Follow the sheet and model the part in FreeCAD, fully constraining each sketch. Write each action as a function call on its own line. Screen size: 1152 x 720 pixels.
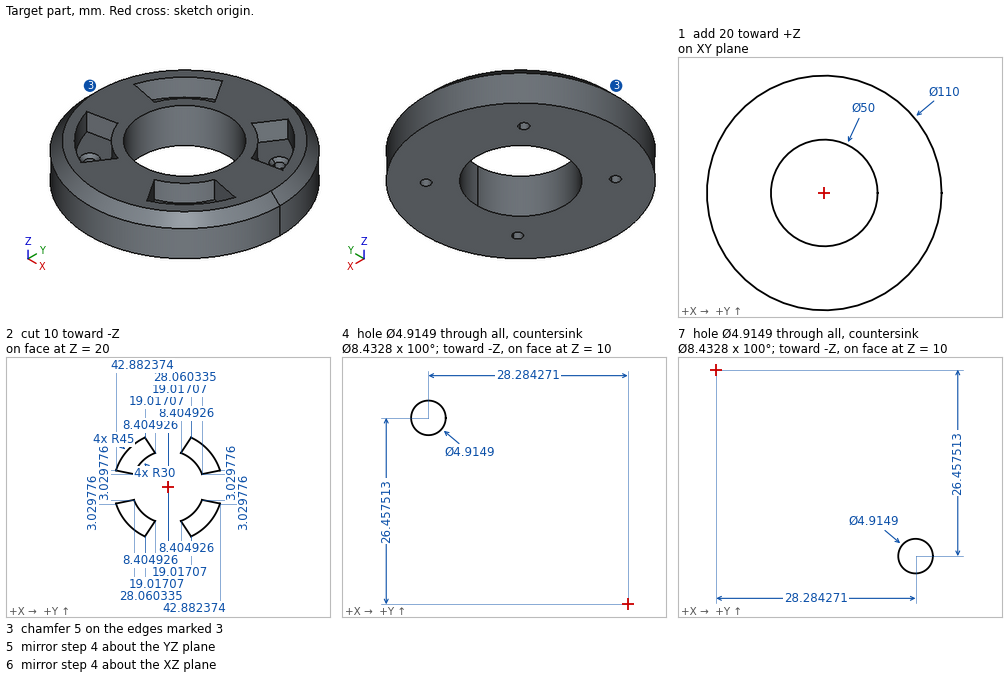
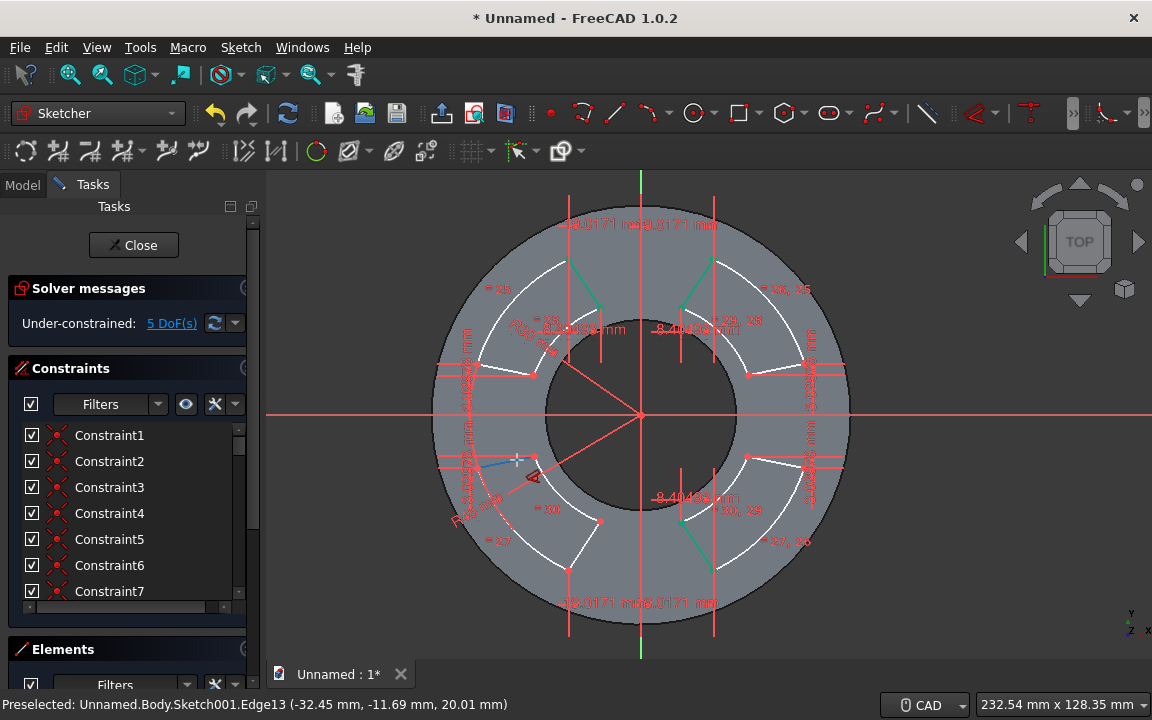
scroll(578, 556, up, 2)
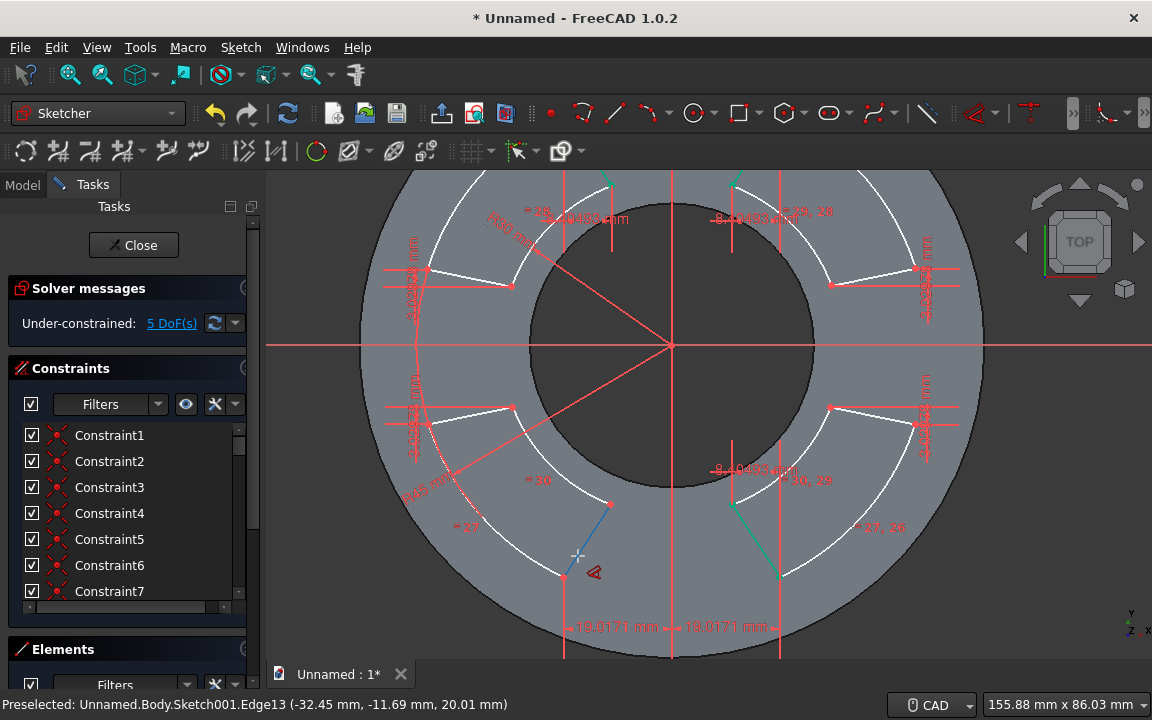
click(578, 555)
click(587, 471)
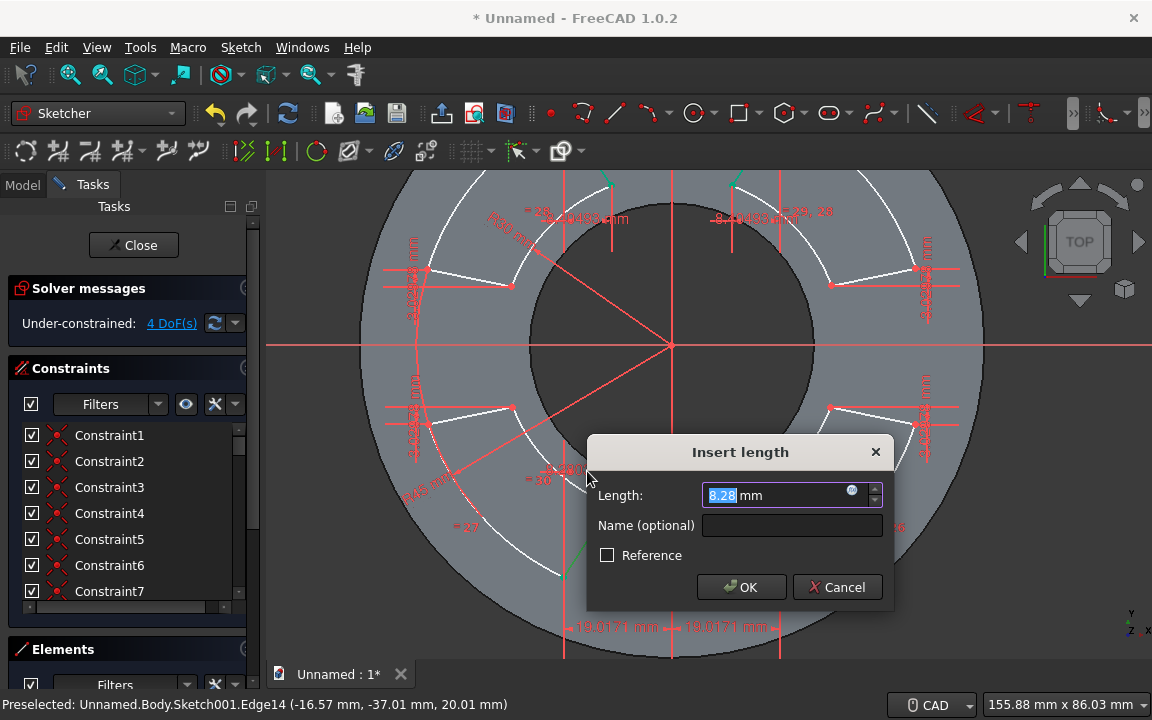
text(8.404926)
key(Return)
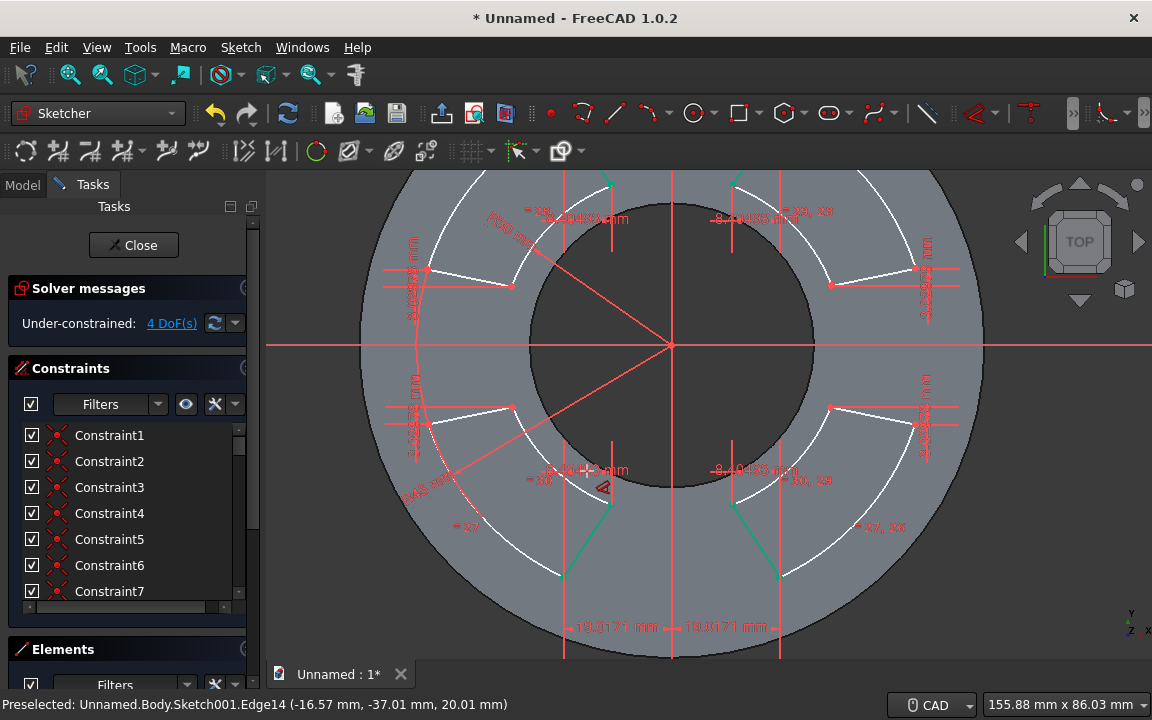
click(428, 270)
click(550, 379)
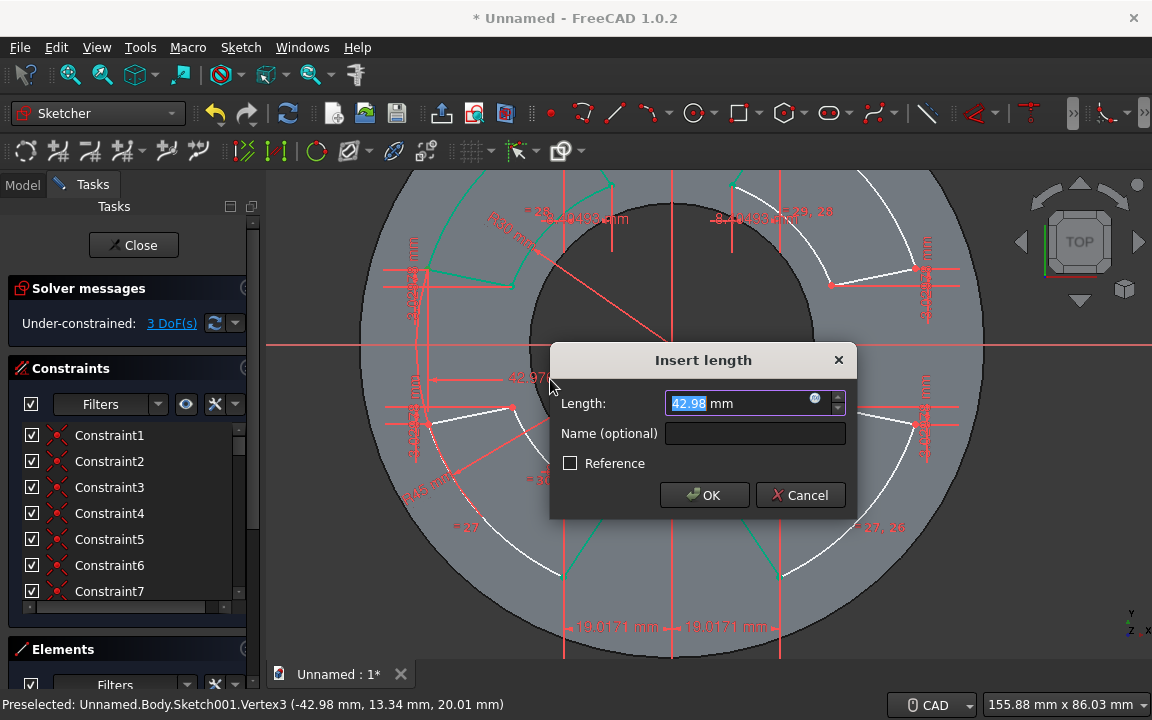
text(42.882374)
key(Return)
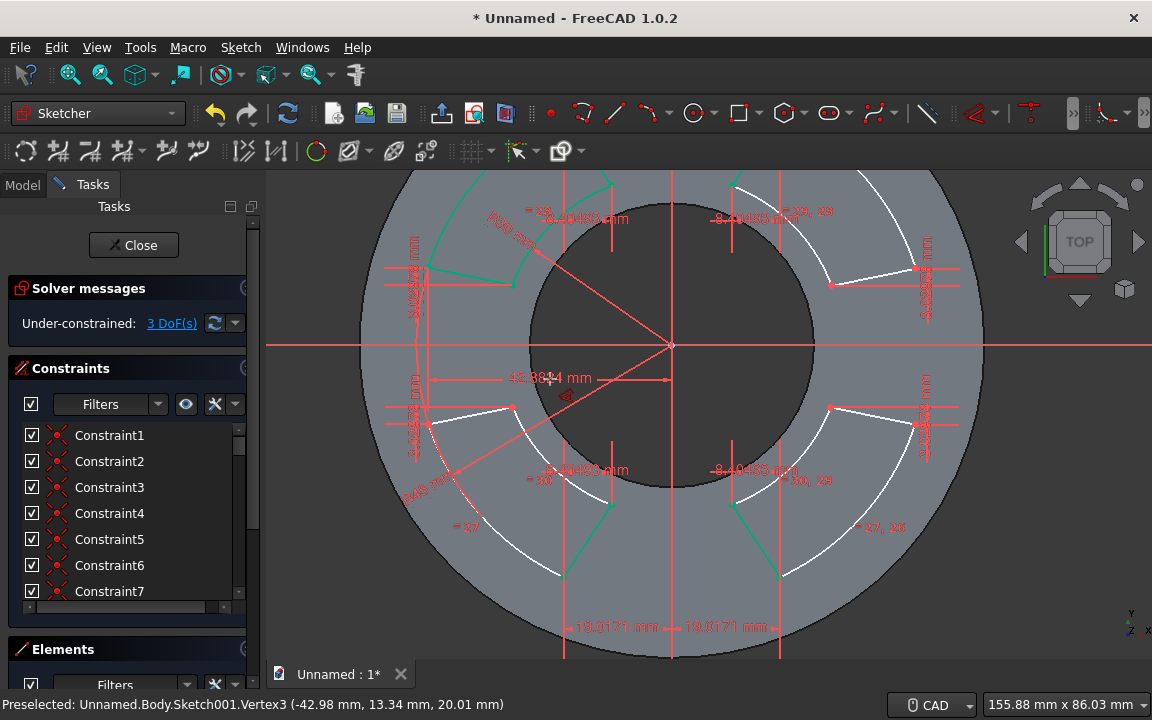
click(832, 286)
click(752, 252)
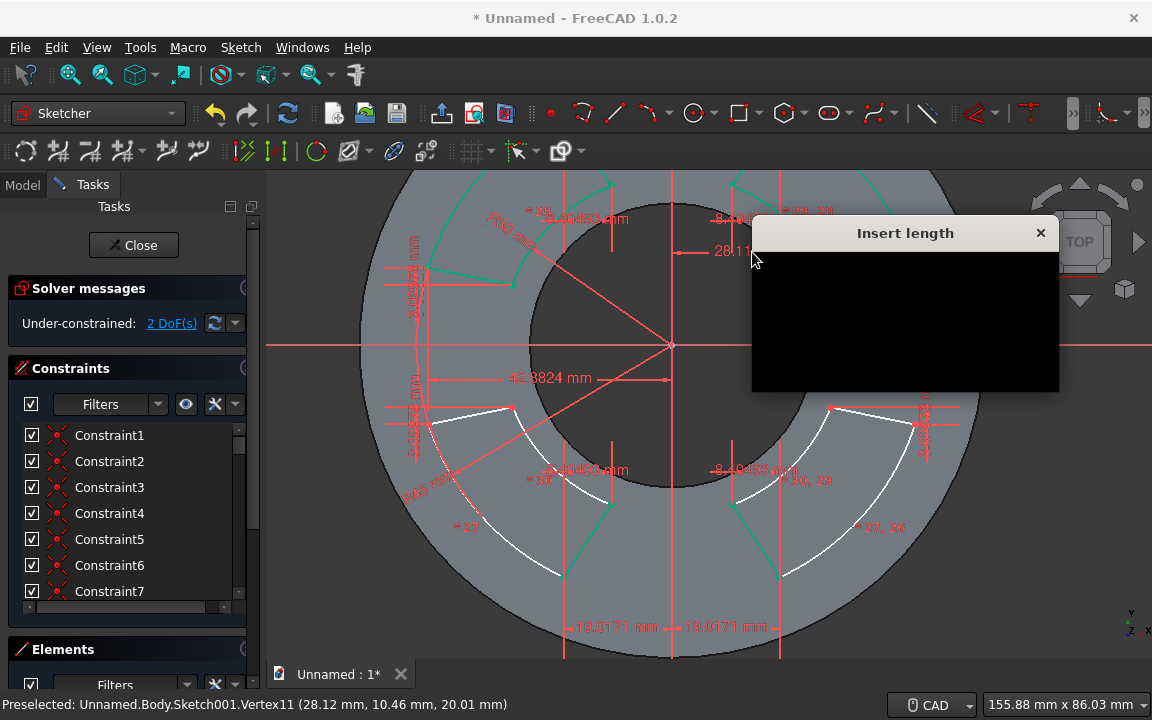
text(28.060335)
key(Return)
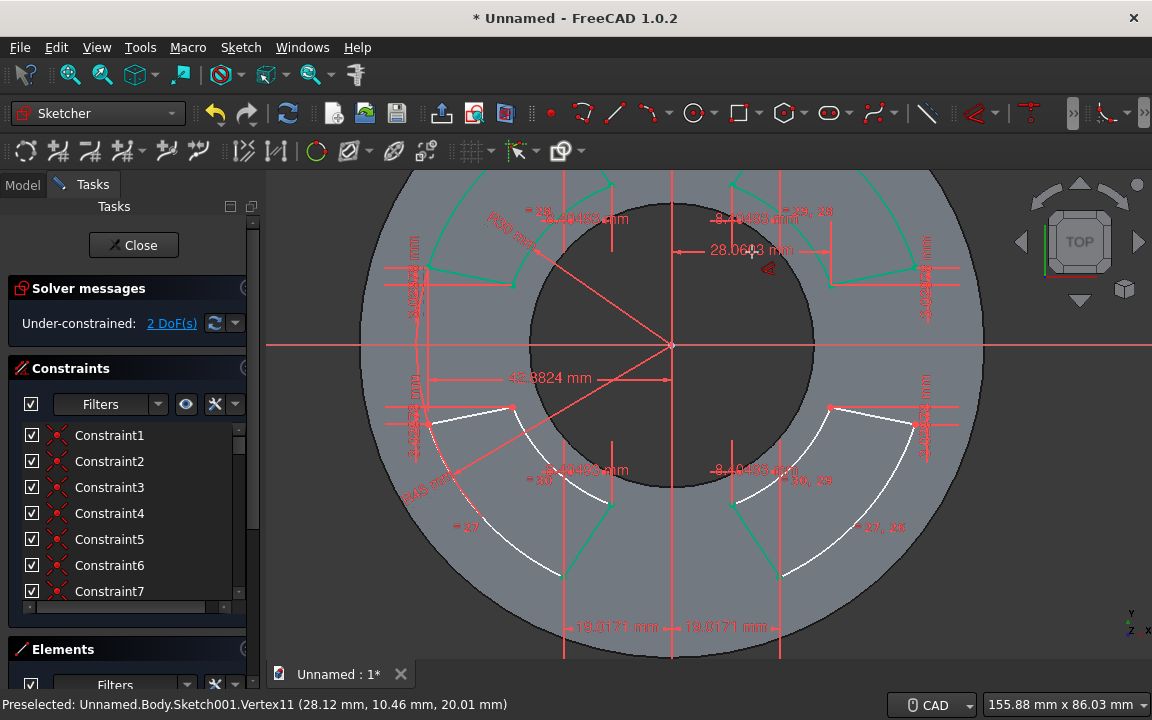
click(915, 425)
click(849, 459)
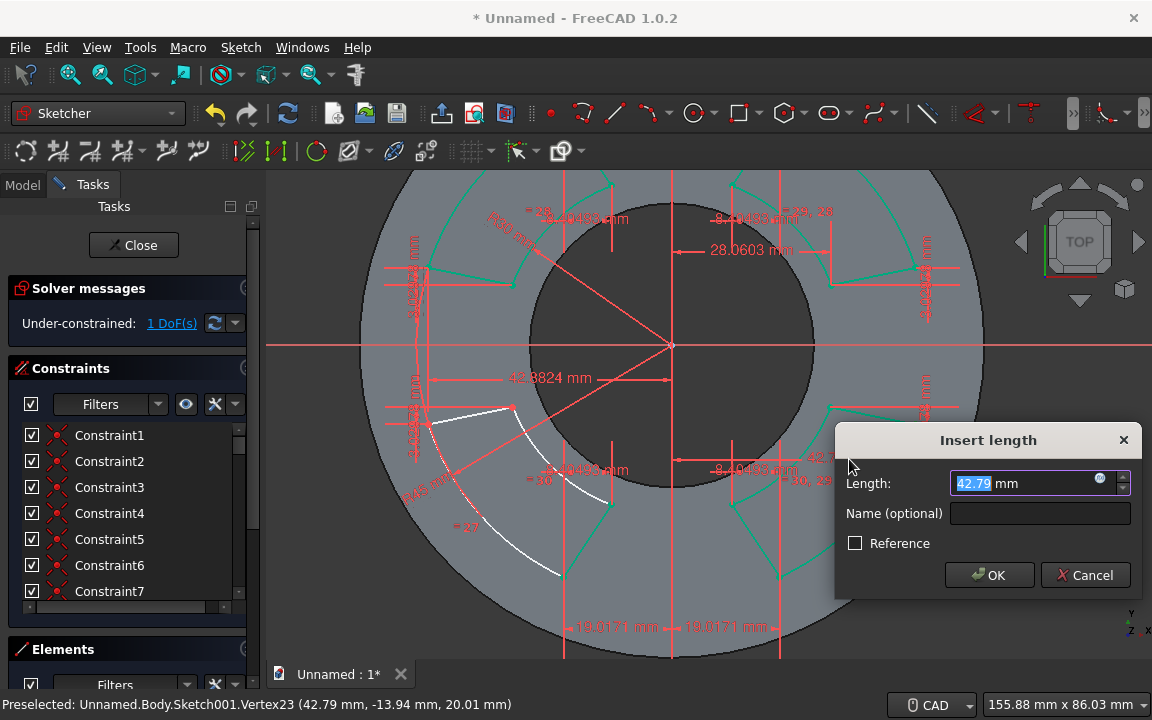
text(42.882374)
key(Return)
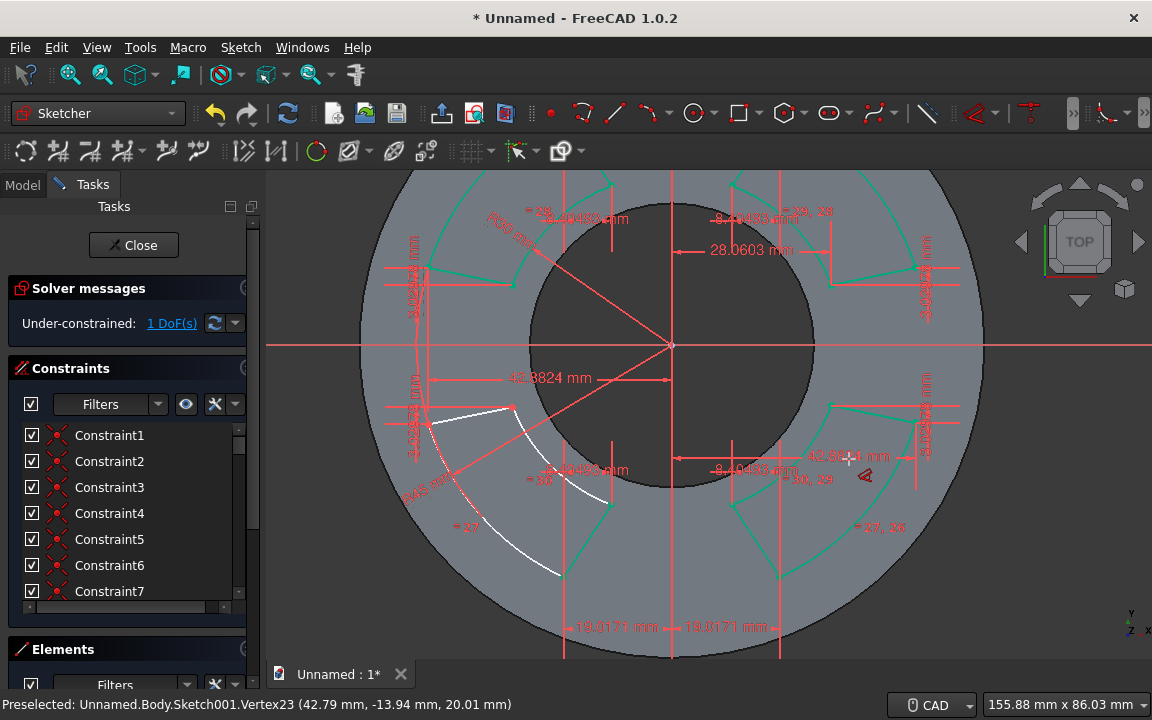
click(513, 407)
click(592, 441)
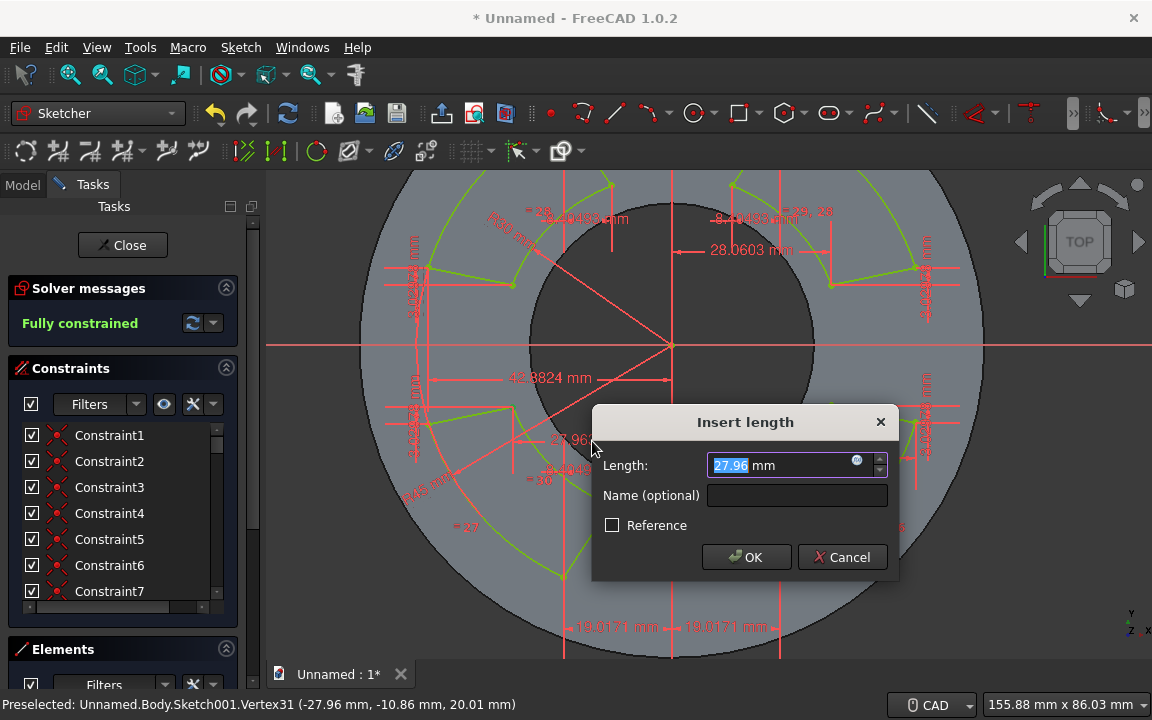
text(28.060335)
key(Return)
key(Escape)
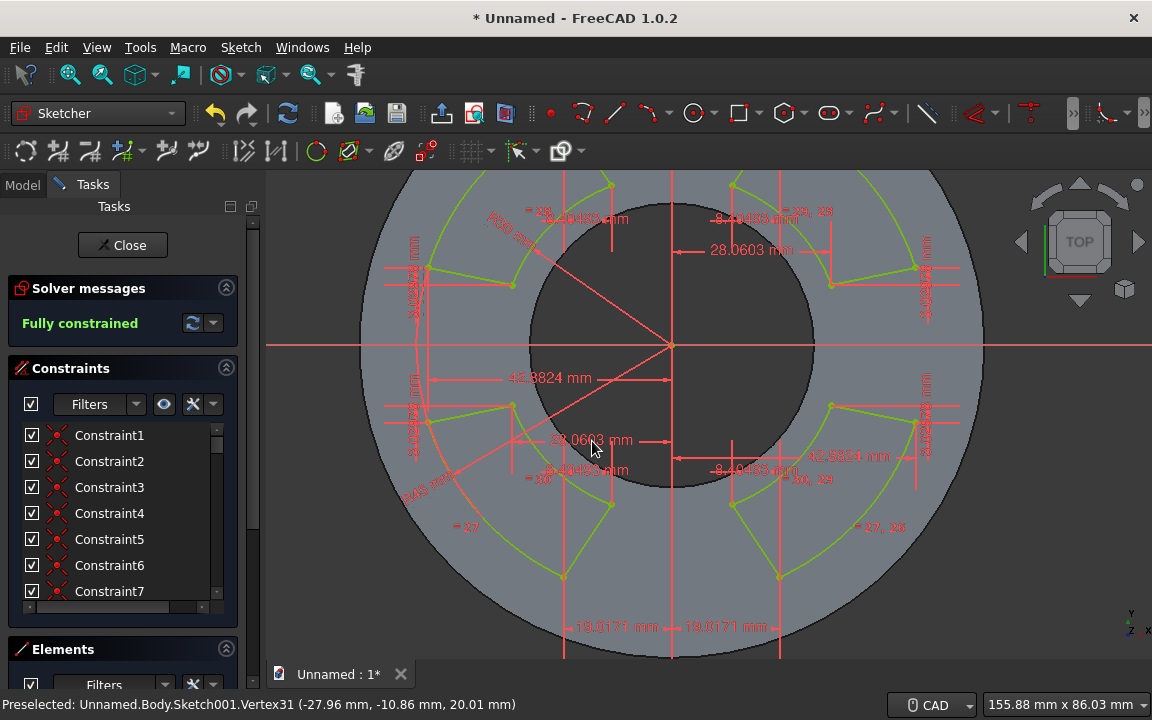
click(123, 245)